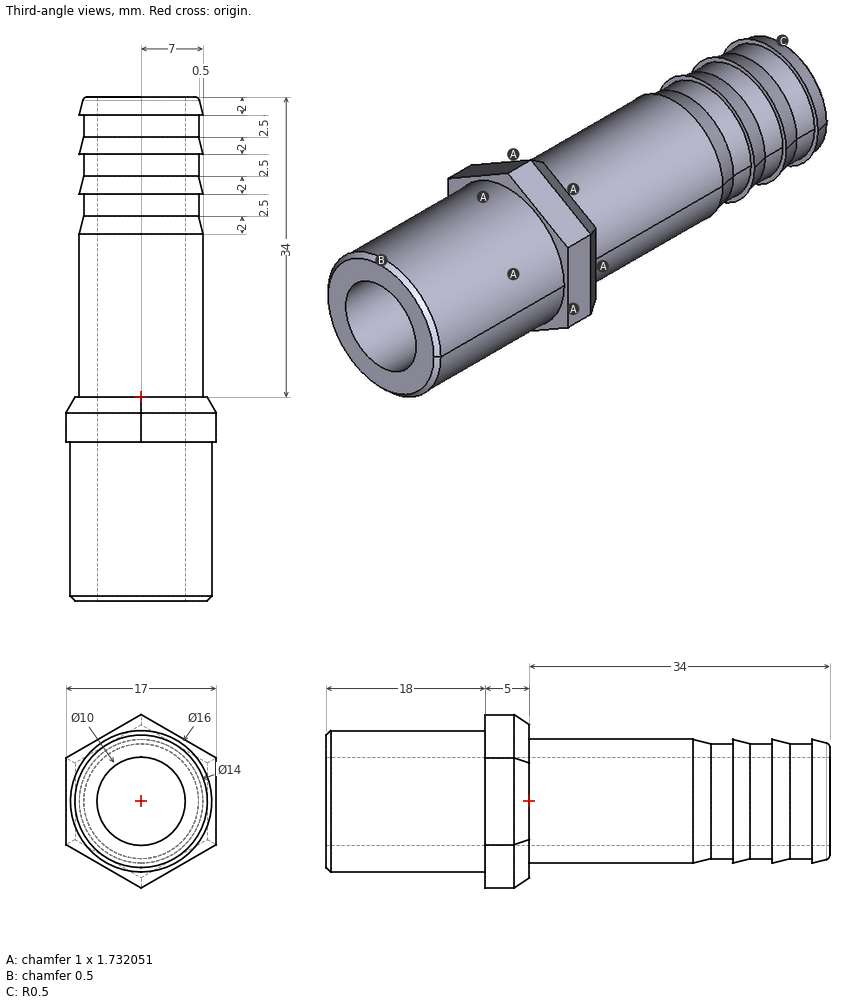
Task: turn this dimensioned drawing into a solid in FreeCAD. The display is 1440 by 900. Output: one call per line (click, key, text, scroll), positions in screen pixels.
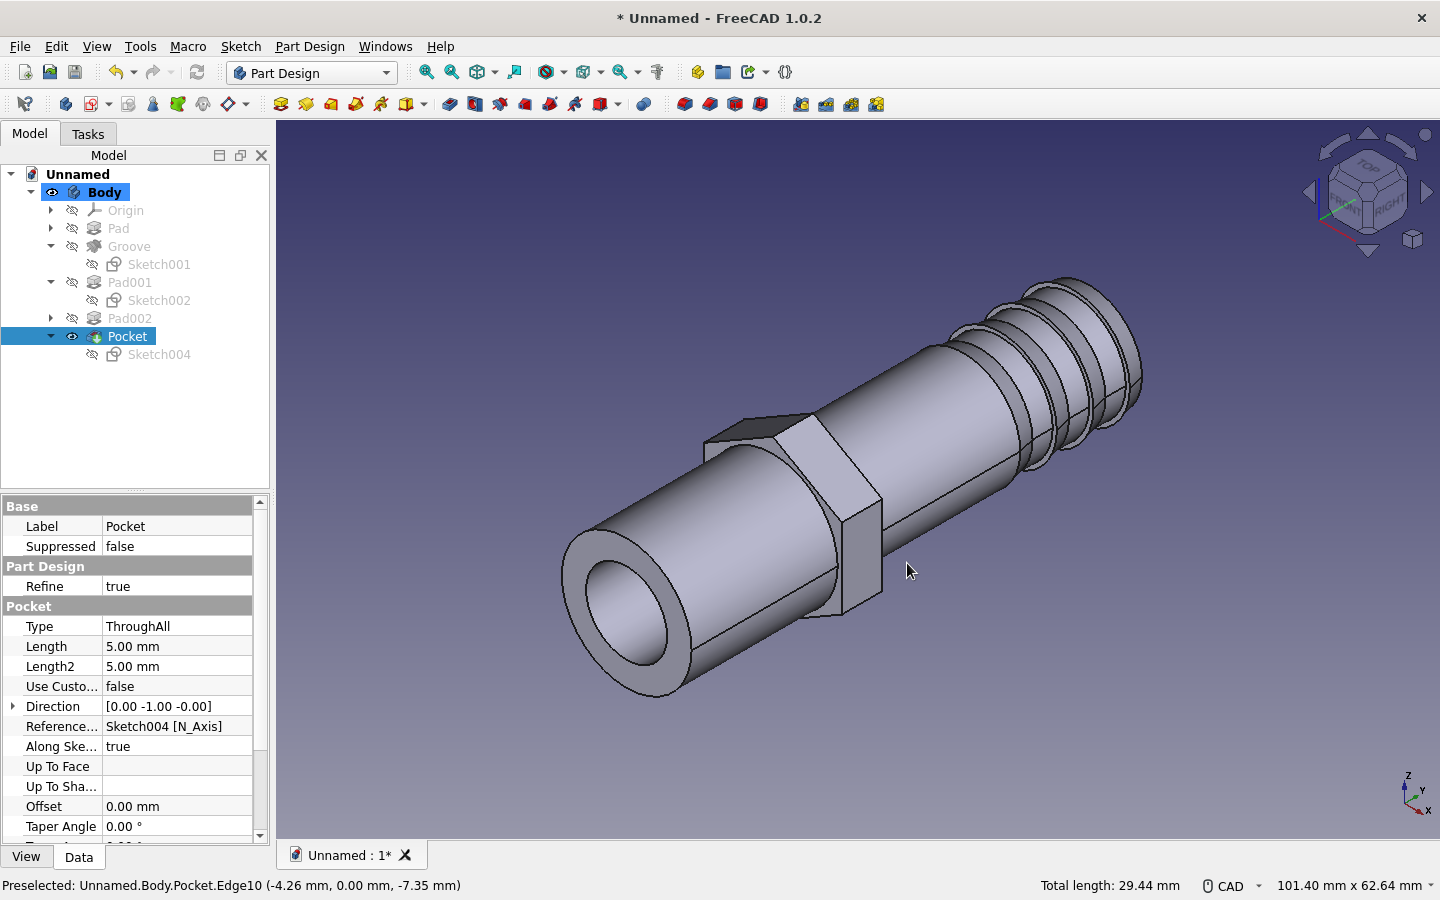
key(2)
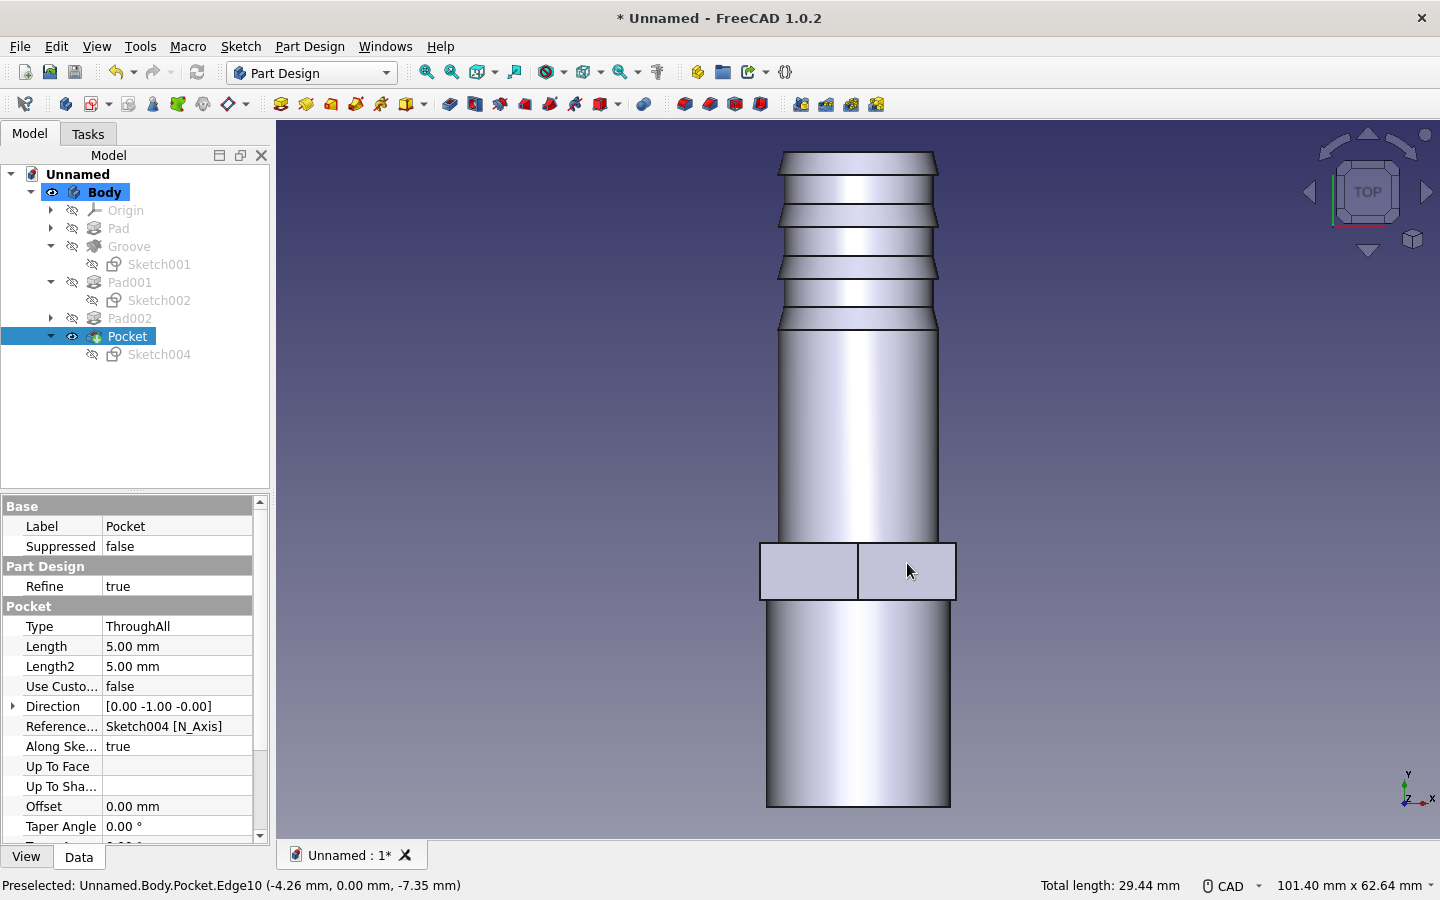
click(907, 542, ctrl)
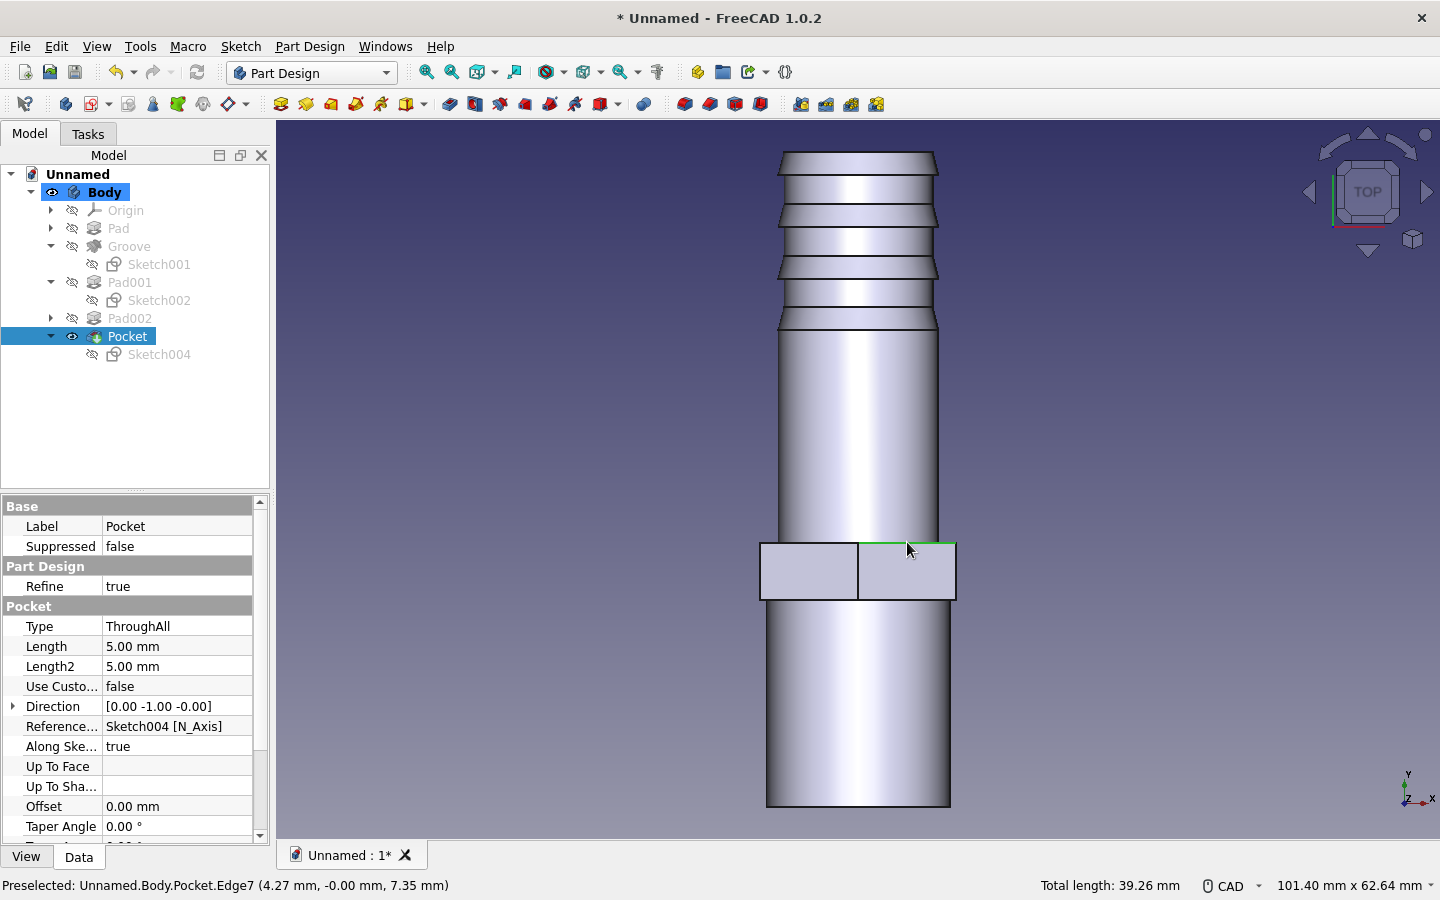
click(809, 542, ctrl)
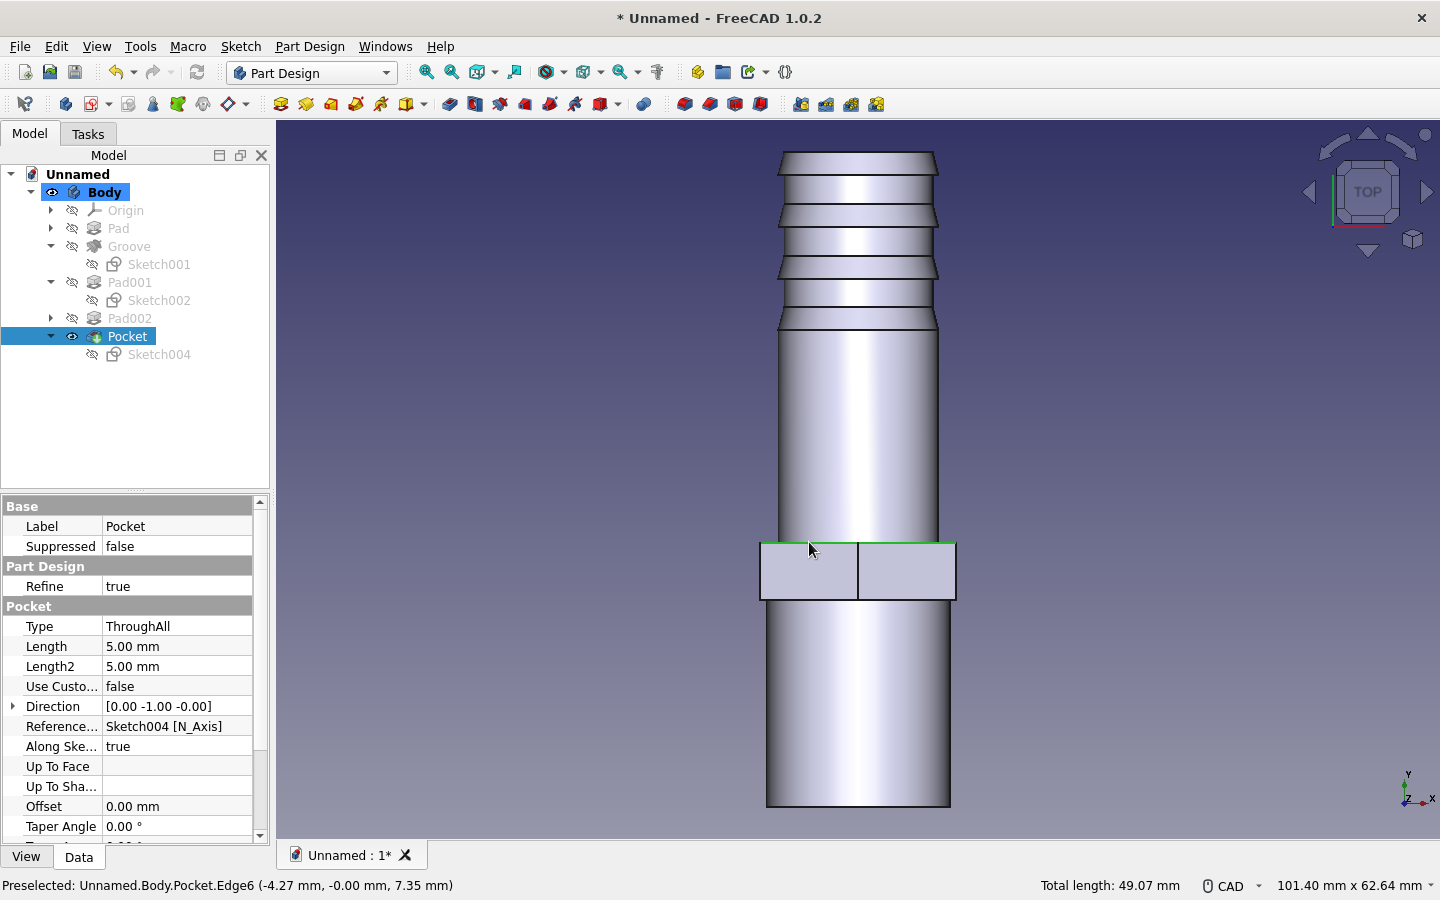
key(1)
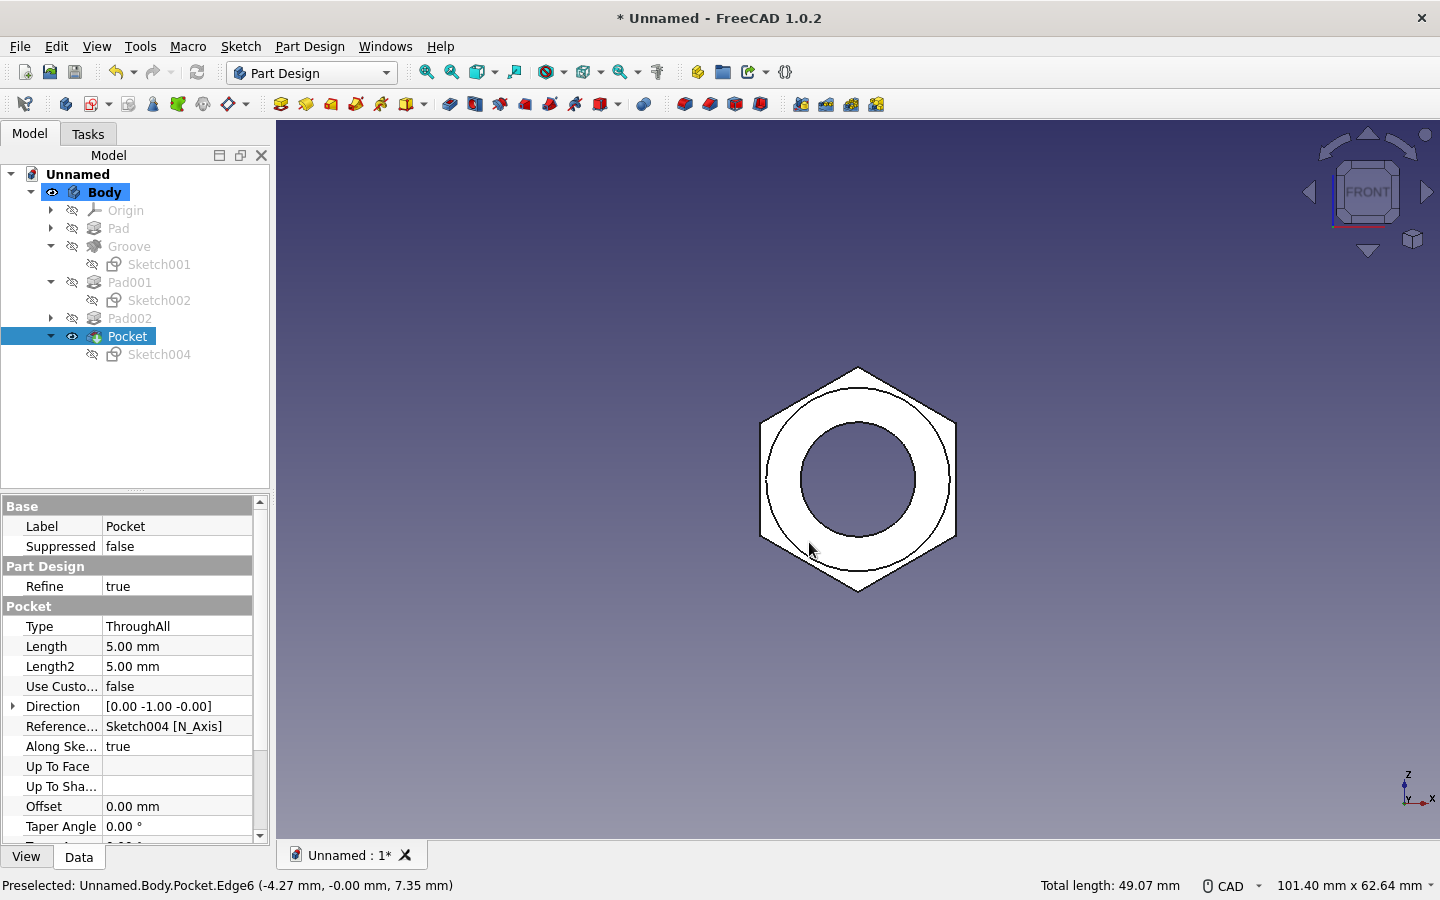
click(427, 72)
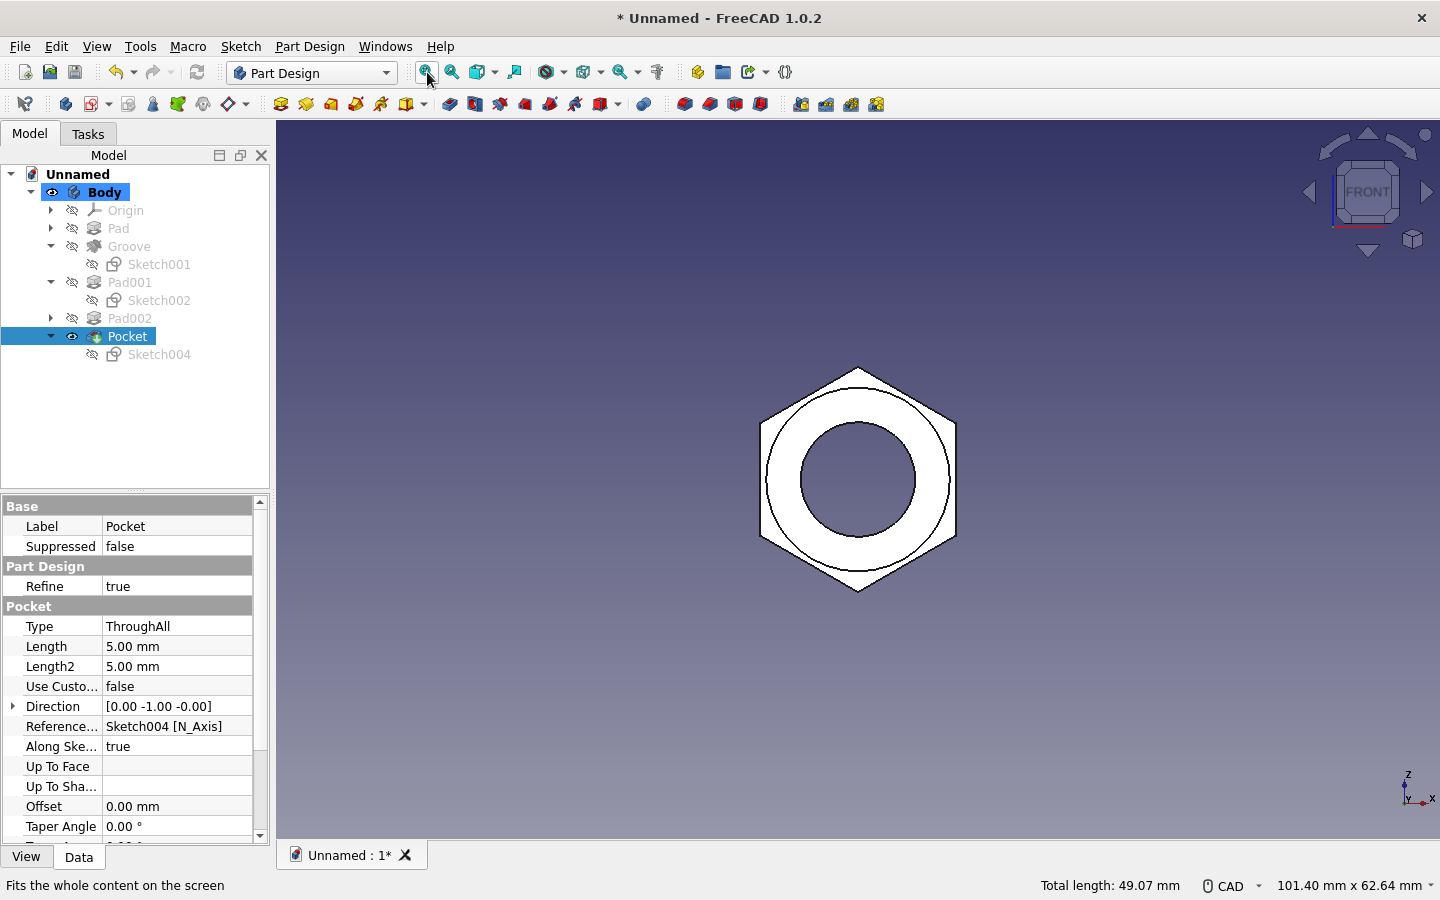
key(3)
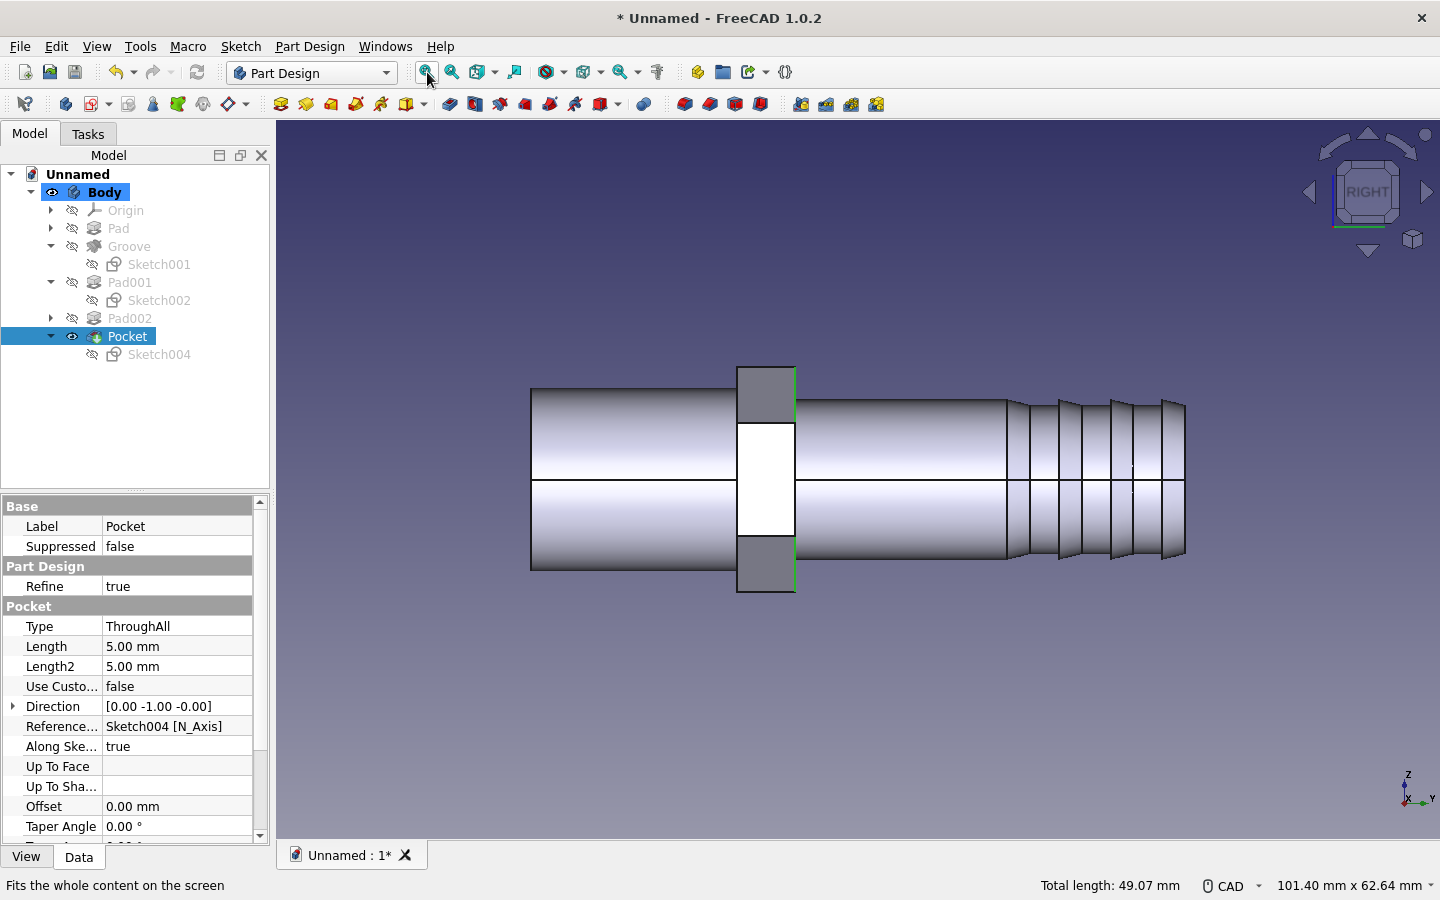
click(795, 478, ctrl)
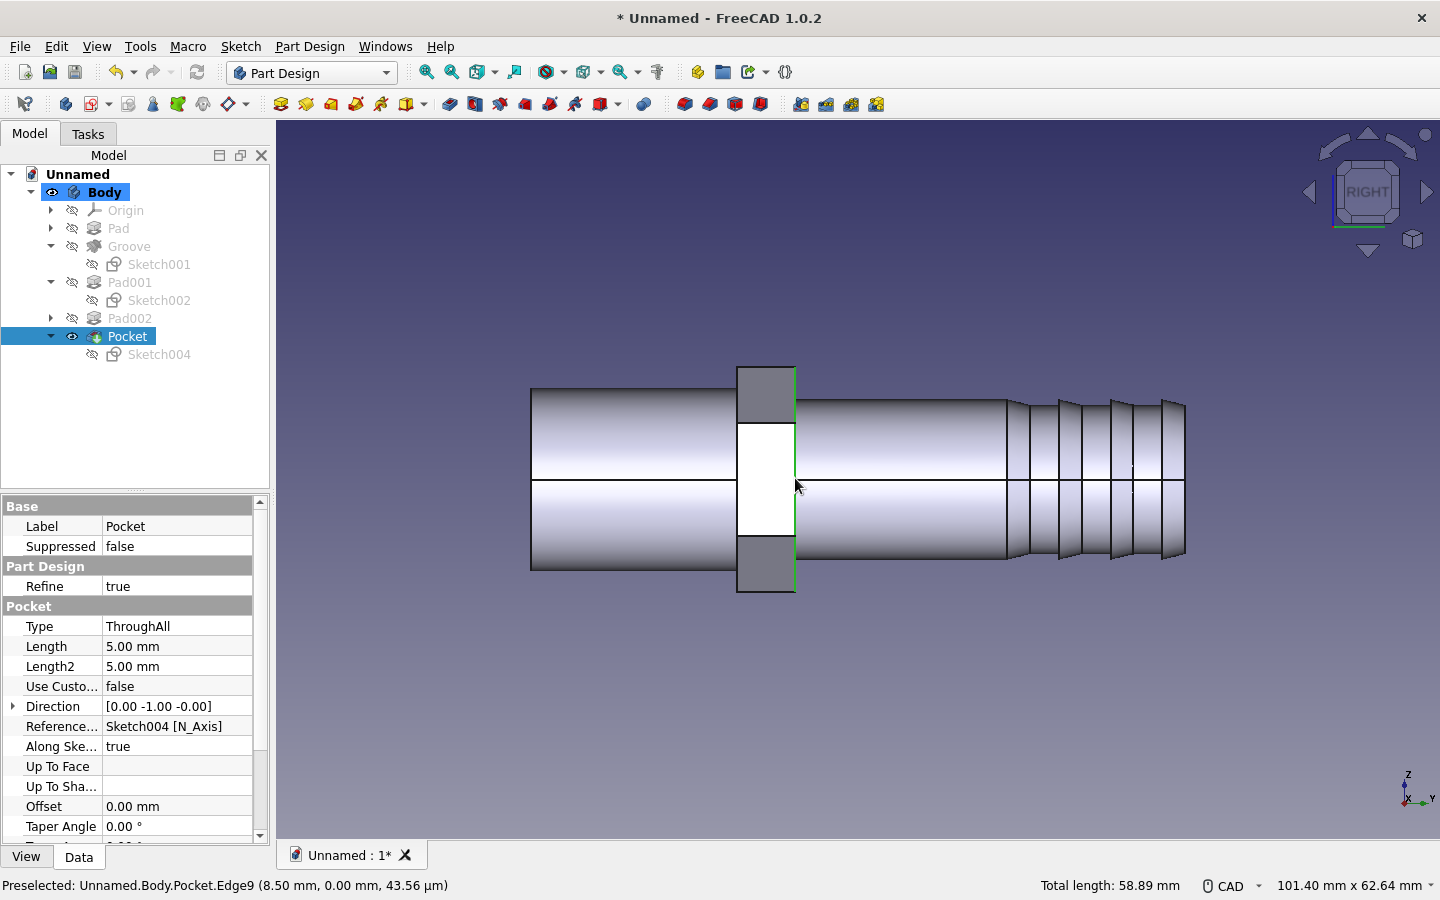
click(710, 104)